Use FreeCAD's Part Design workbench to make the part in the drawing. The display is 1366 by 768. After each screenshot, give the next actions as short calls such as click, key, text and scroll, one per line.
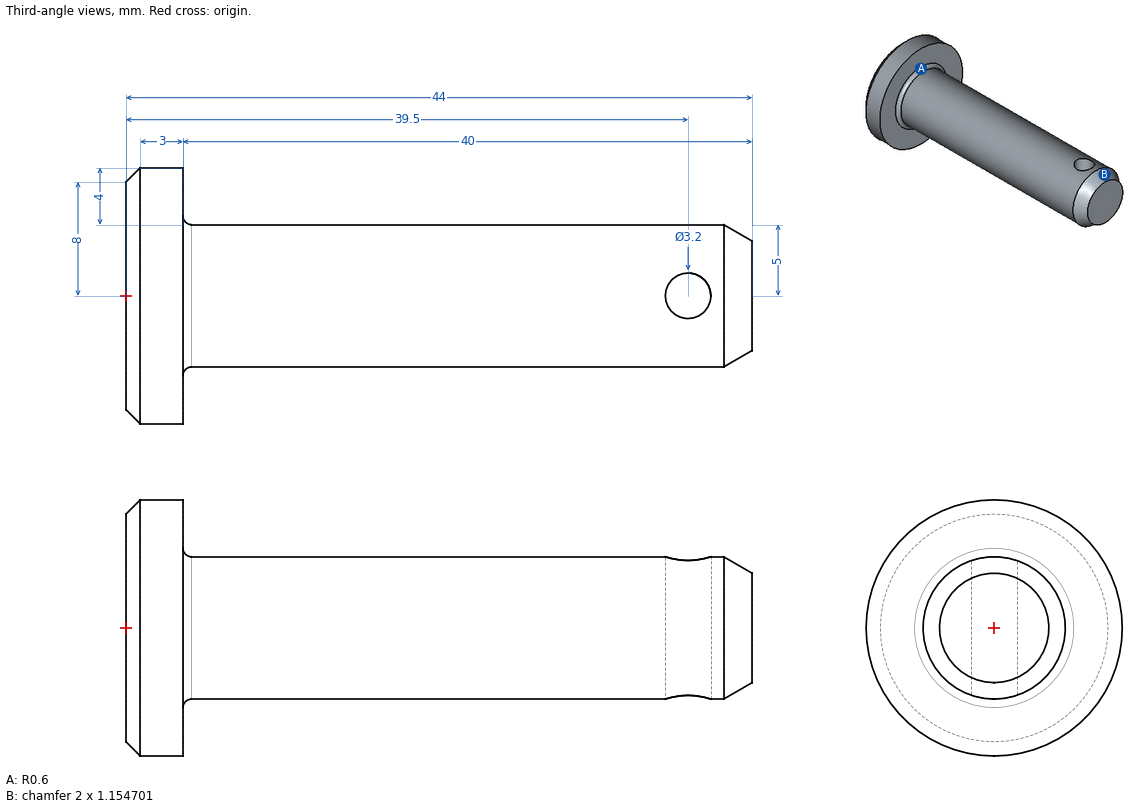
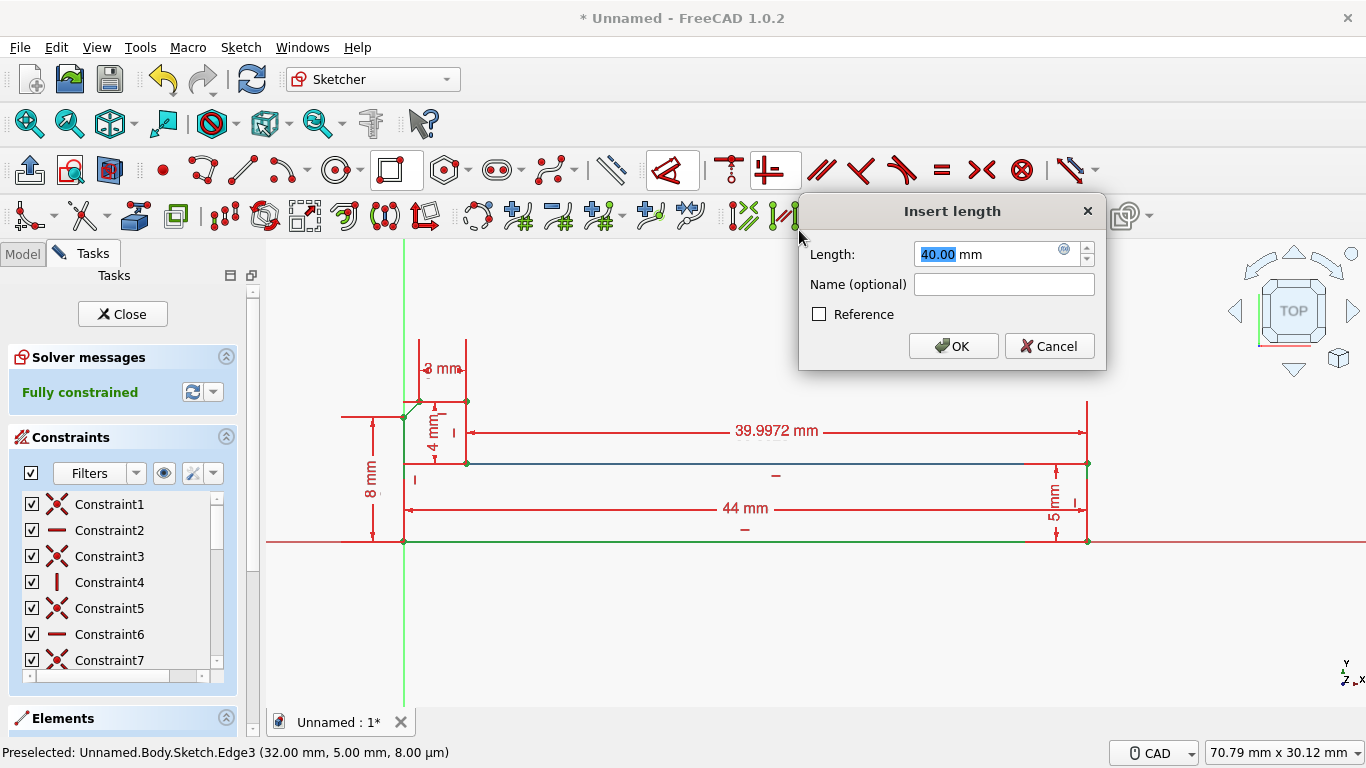
text(40)
key(Return)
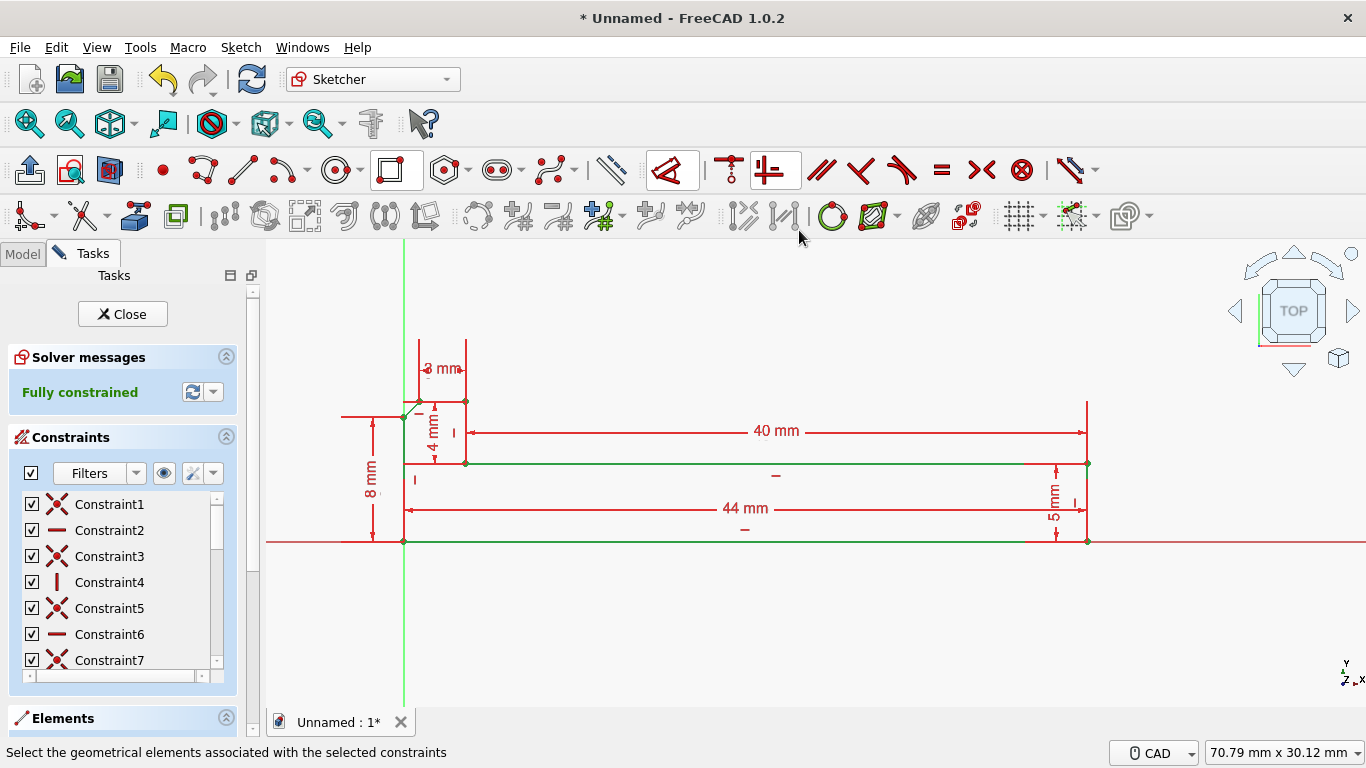
click(123, 314)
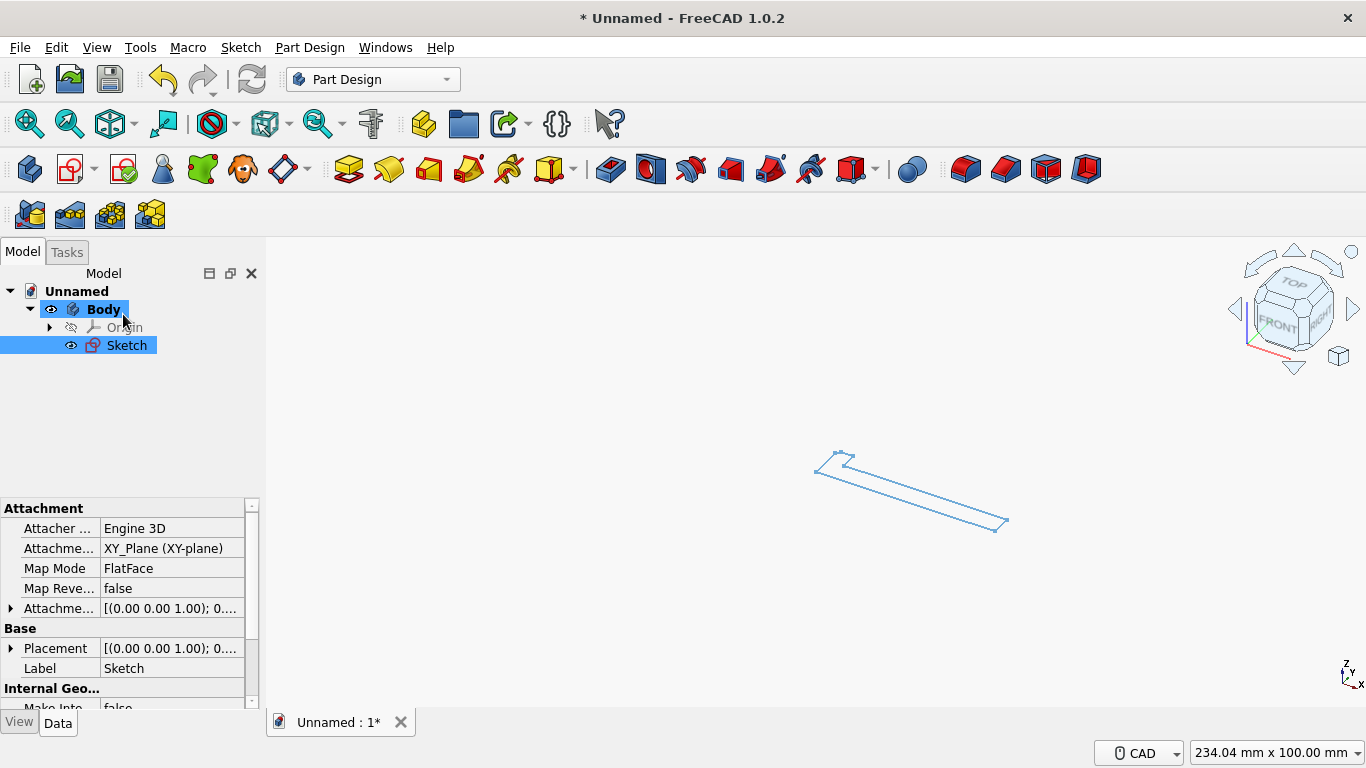
click(390, 170)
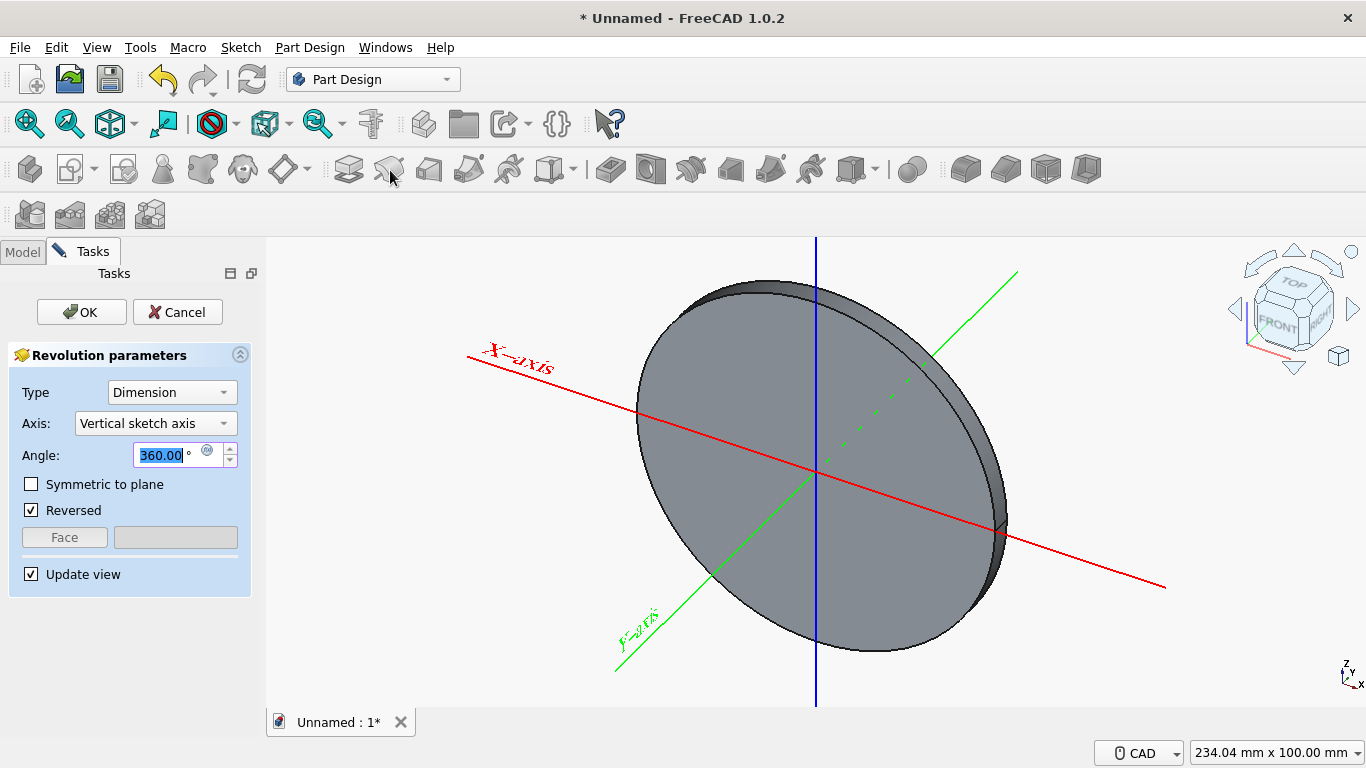
click(156, 424)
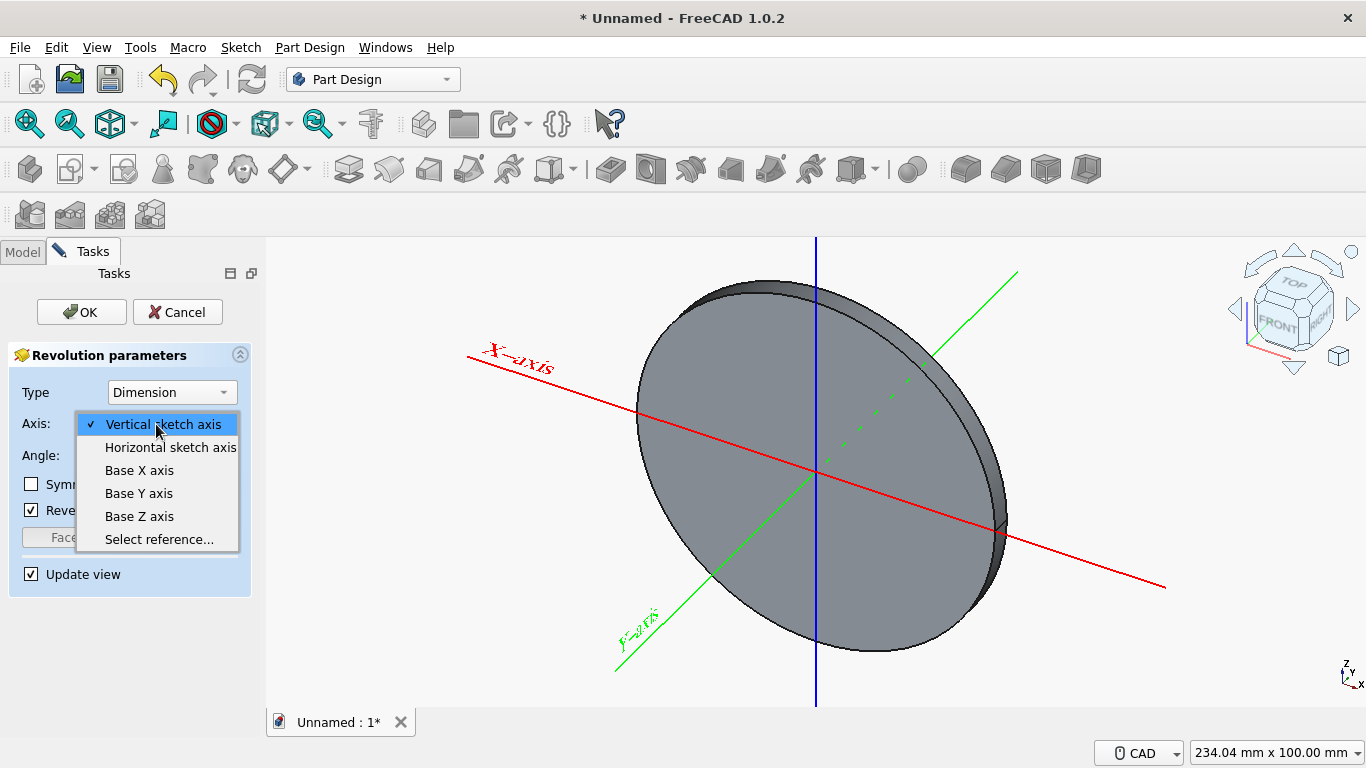
click(156, 448)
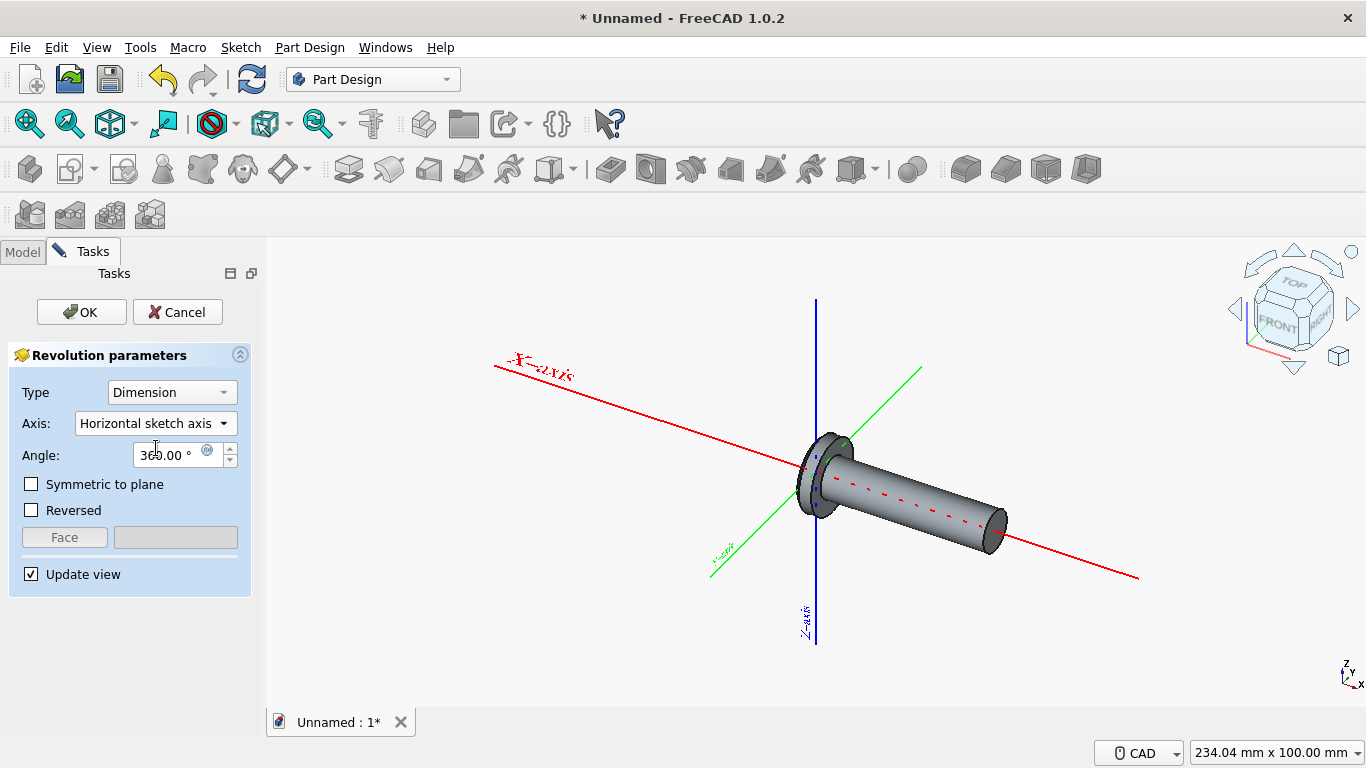
click(82, 312)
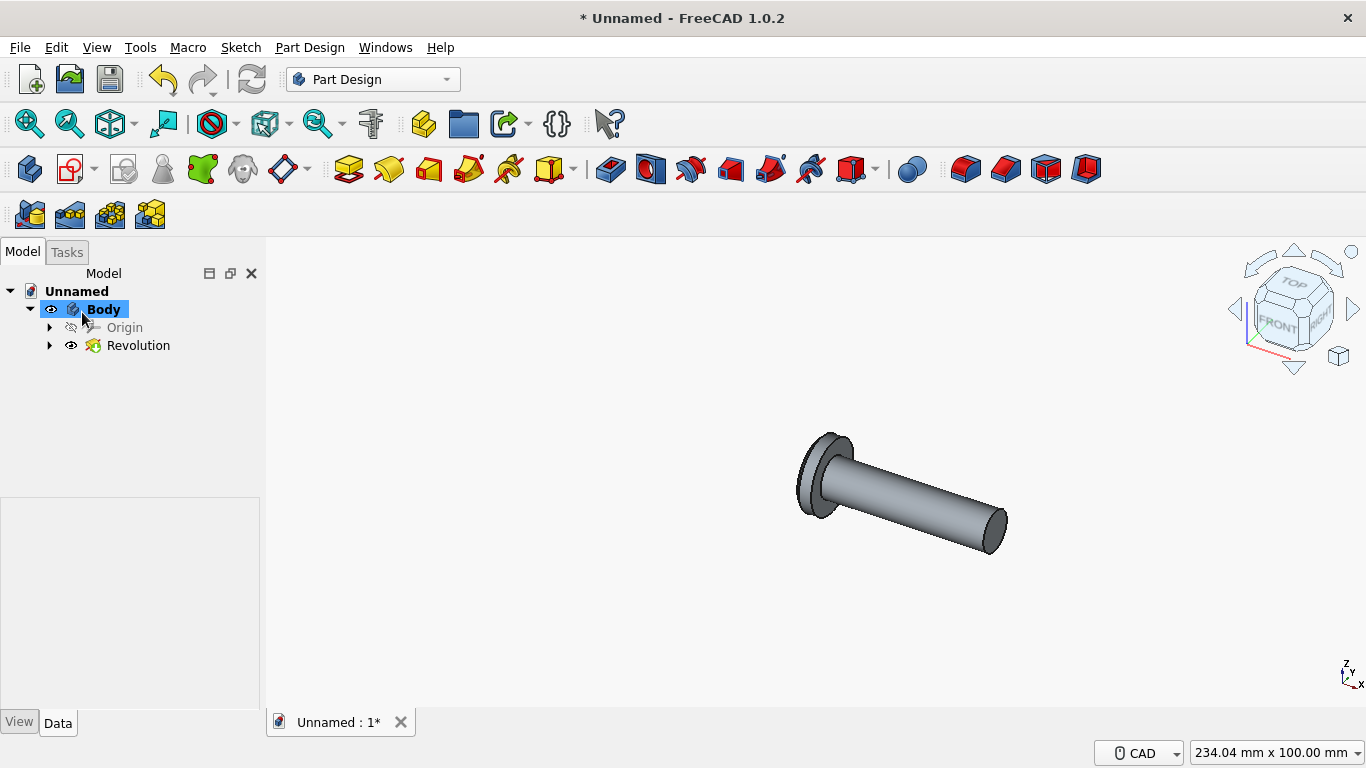
click(30, 124)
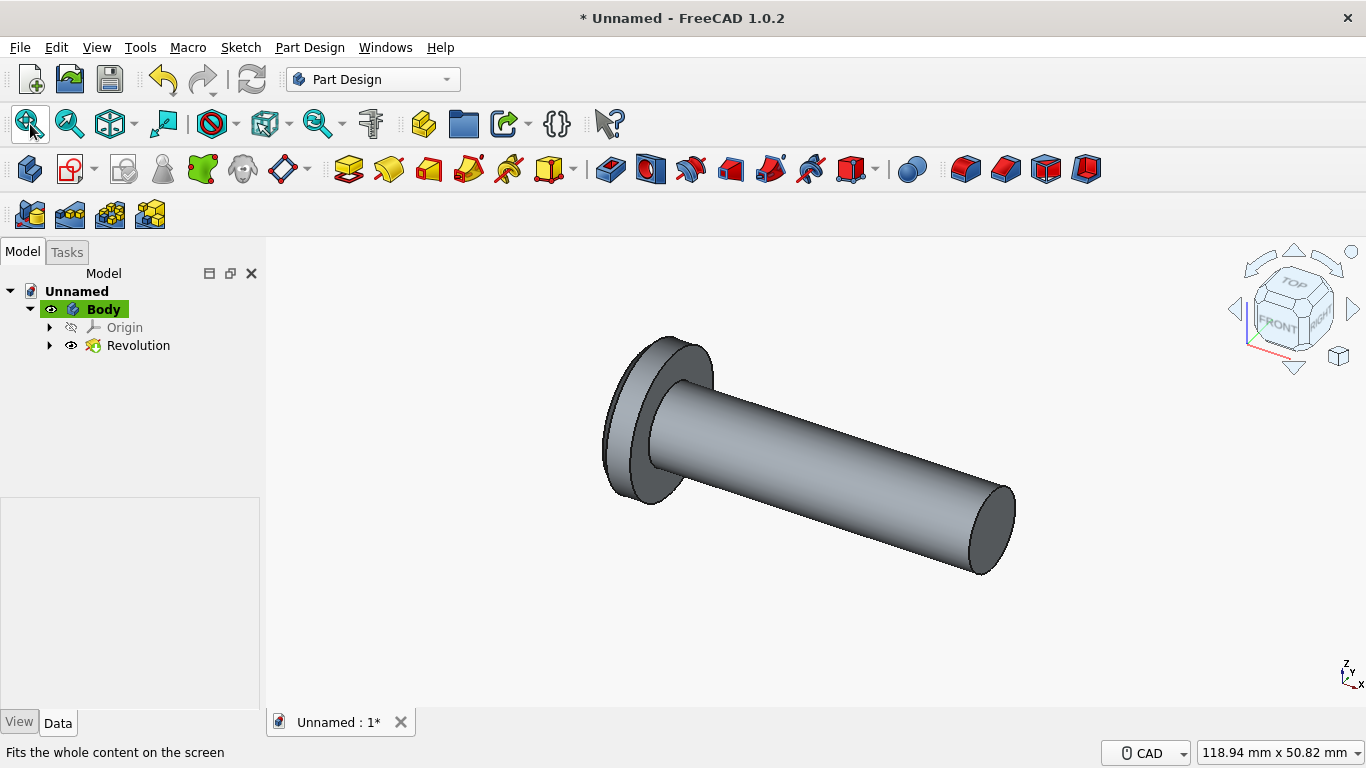
click(70, 170)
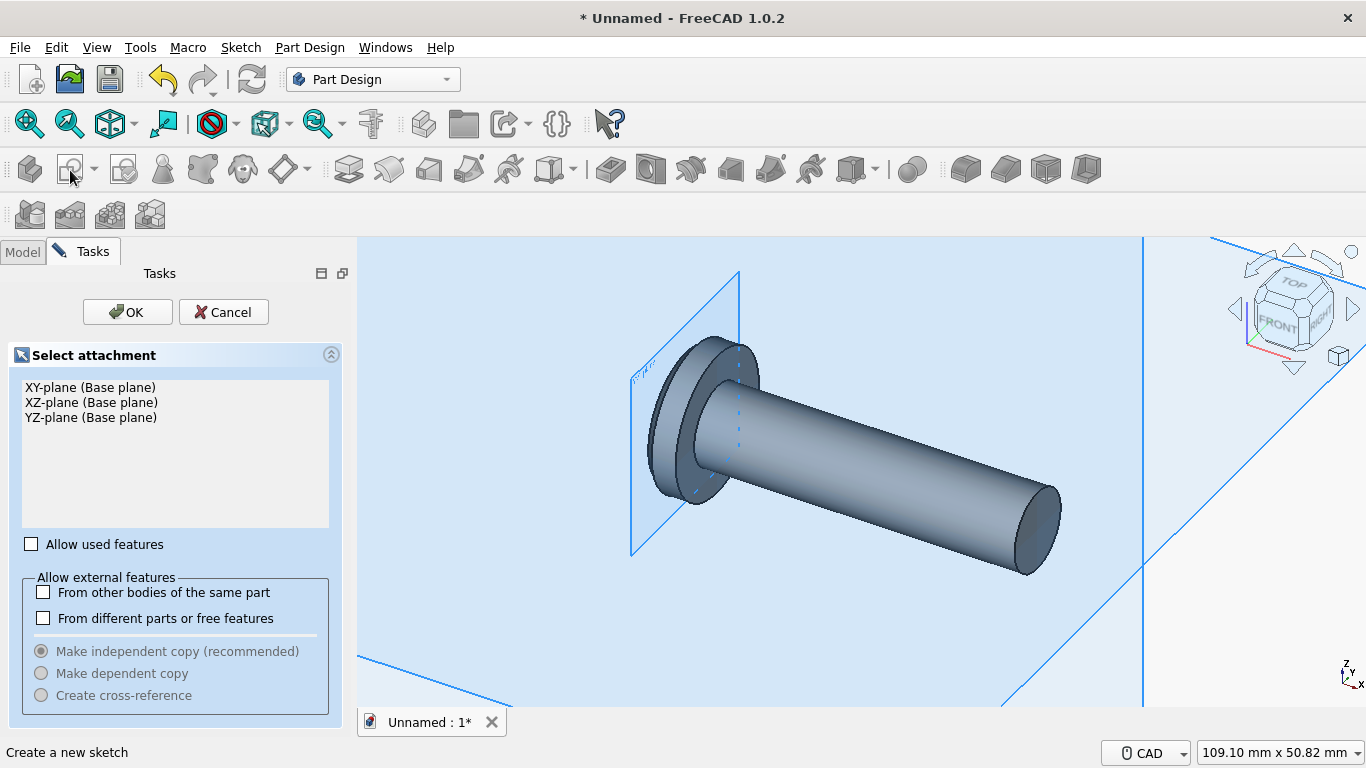
click(82, 388)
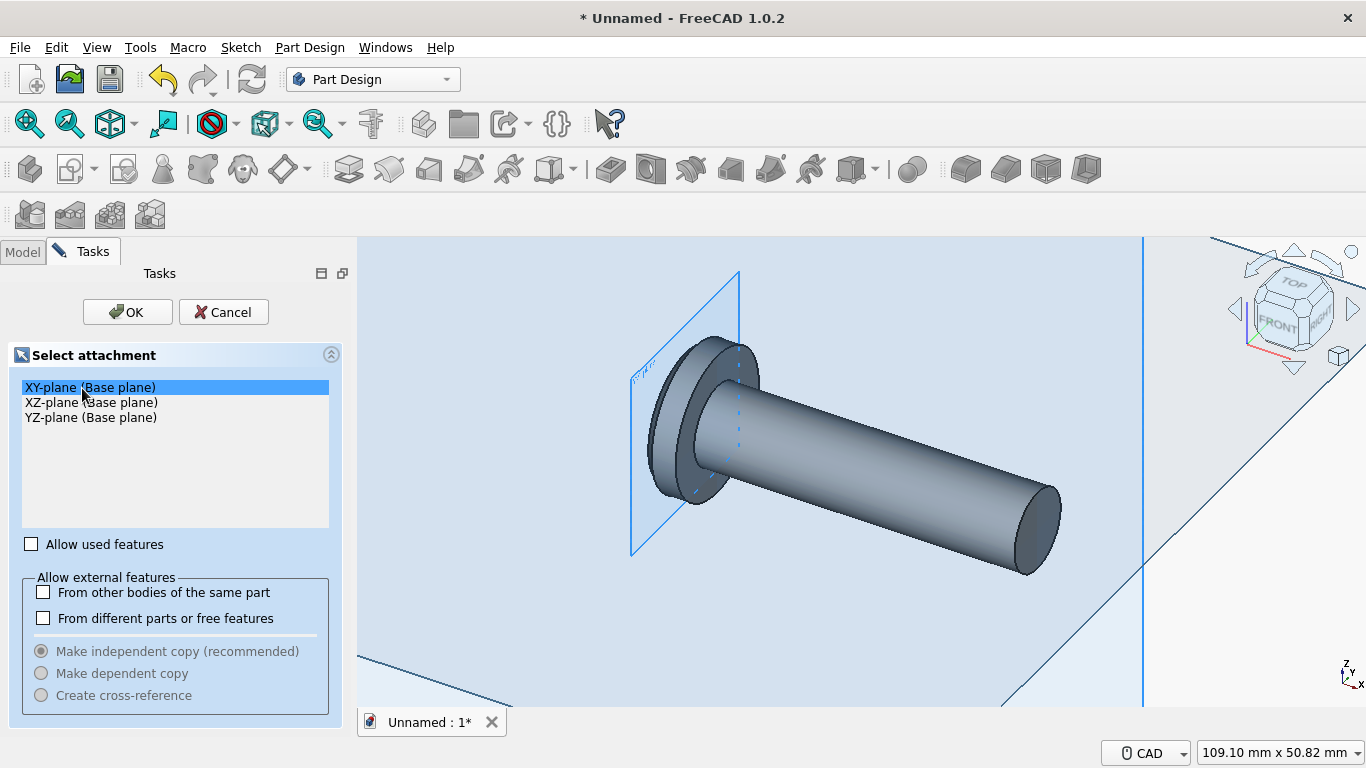
click(128, 312)